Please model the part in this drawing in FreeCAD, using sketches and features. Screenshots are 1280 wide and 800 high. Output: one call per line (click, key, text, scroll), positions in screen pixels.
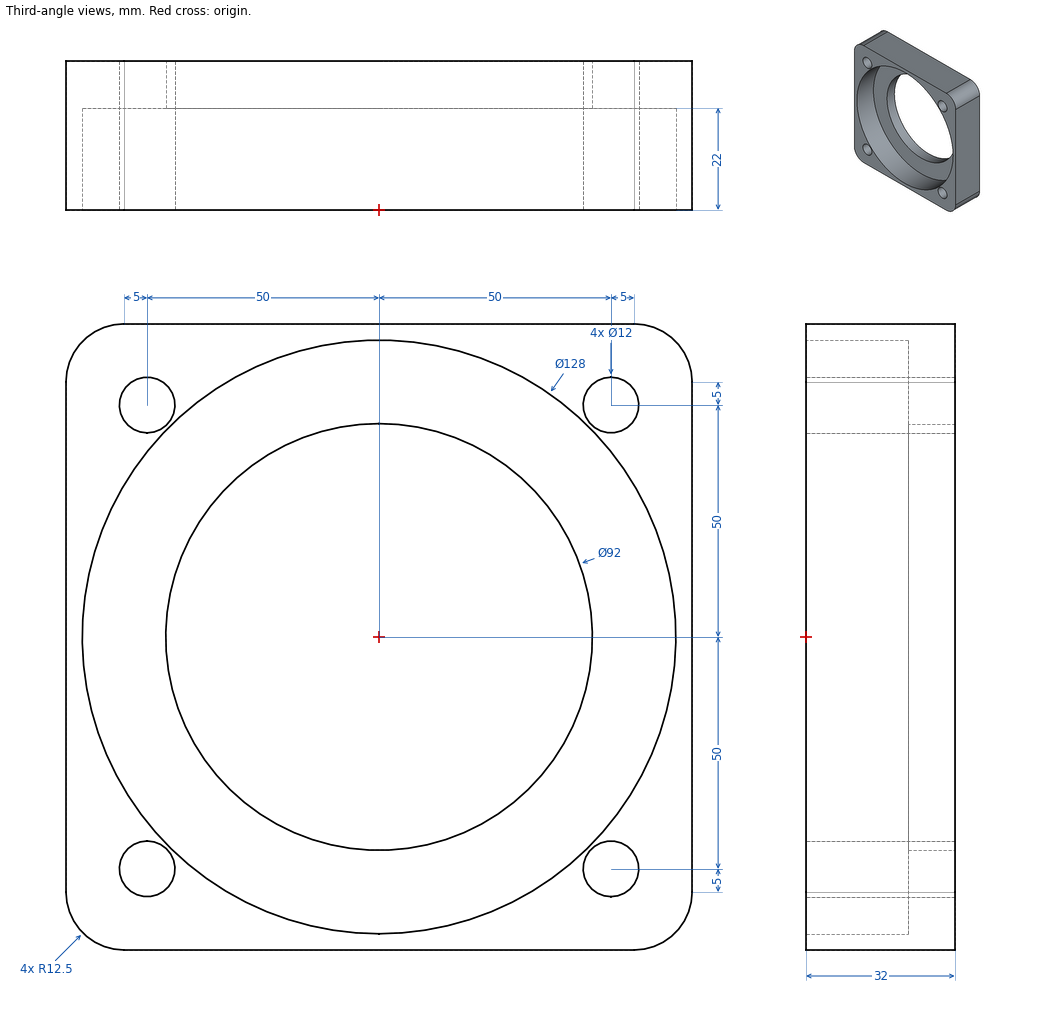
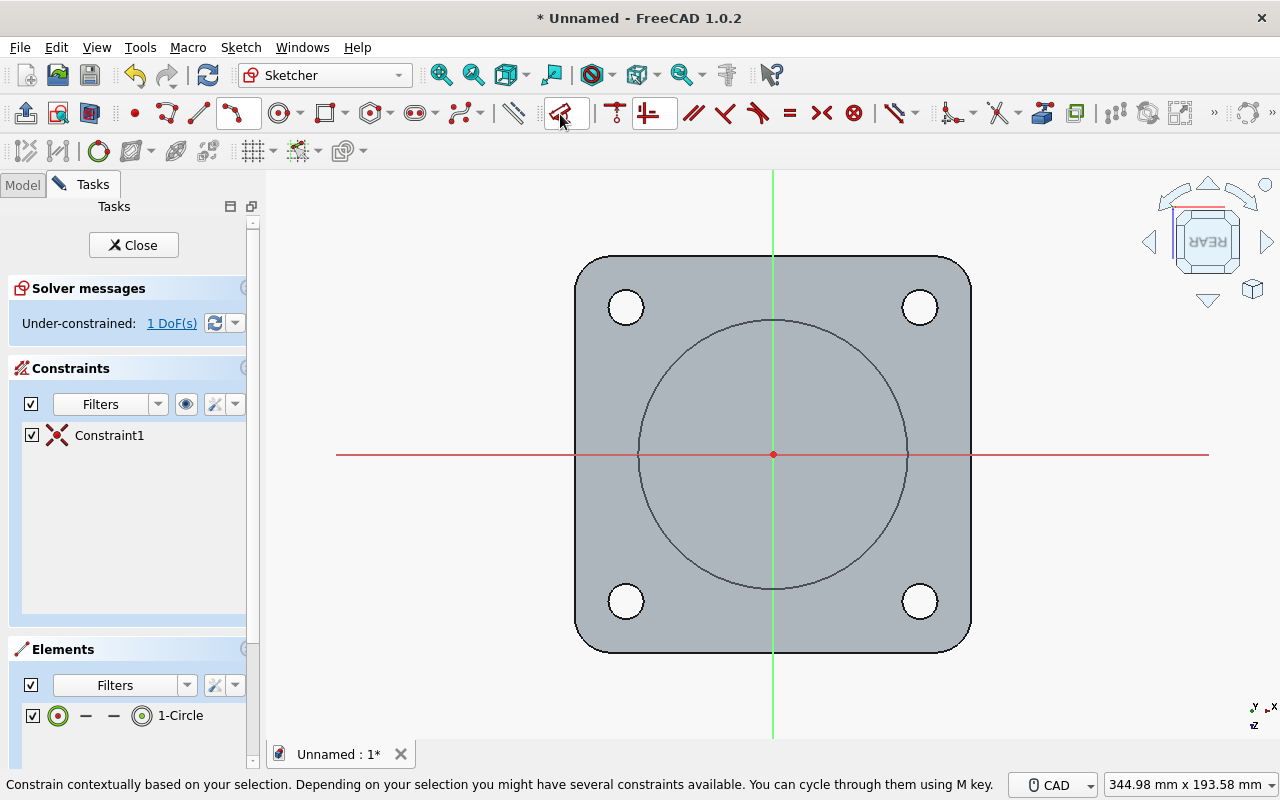
click(868, 359)
click(891, 336)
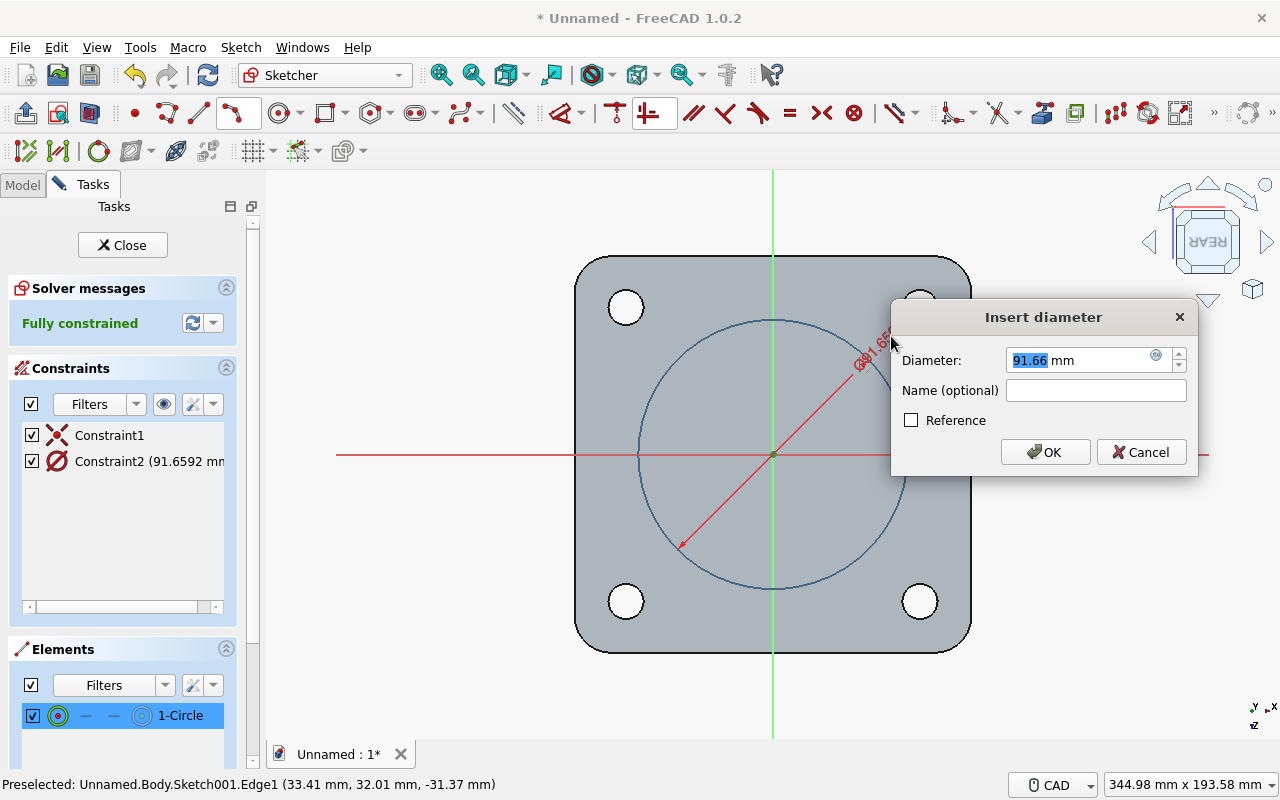
text(92)
key(Return)
key(Escape)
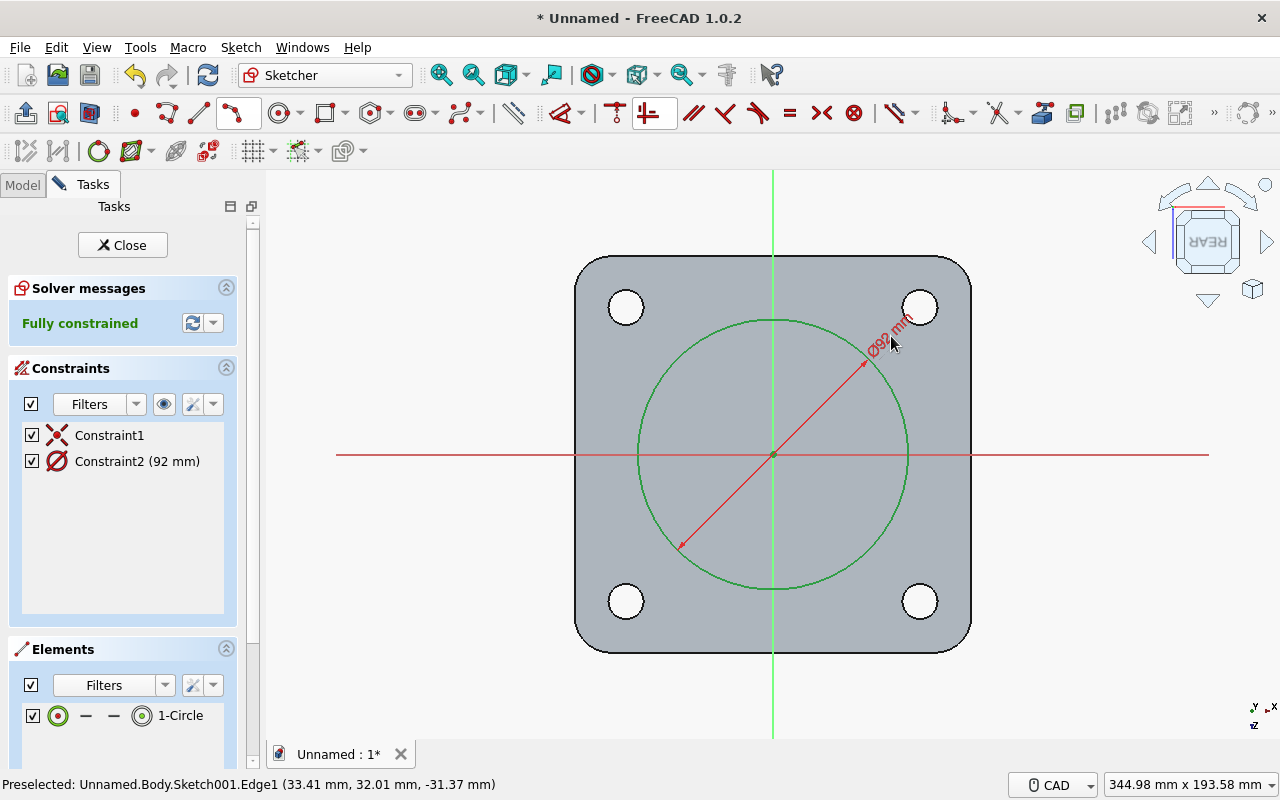
click(123, 245)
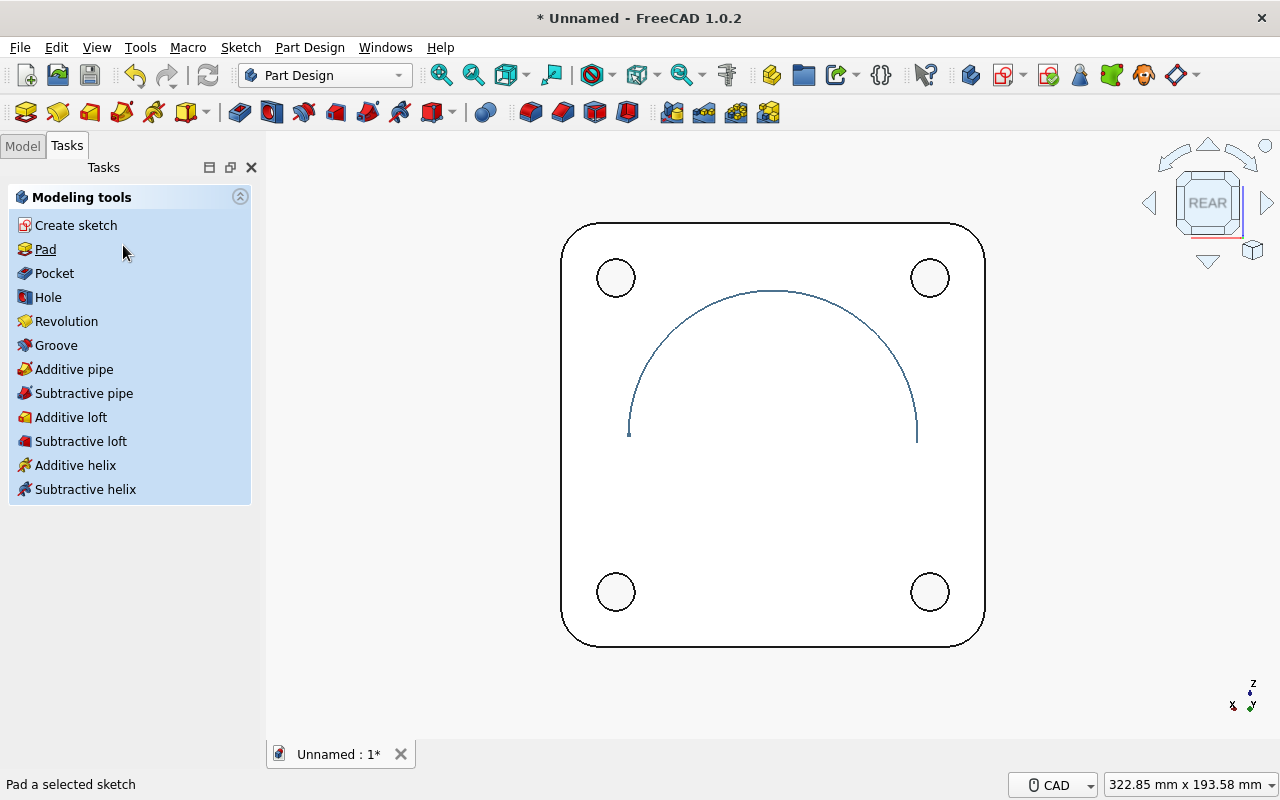
click(240, 112)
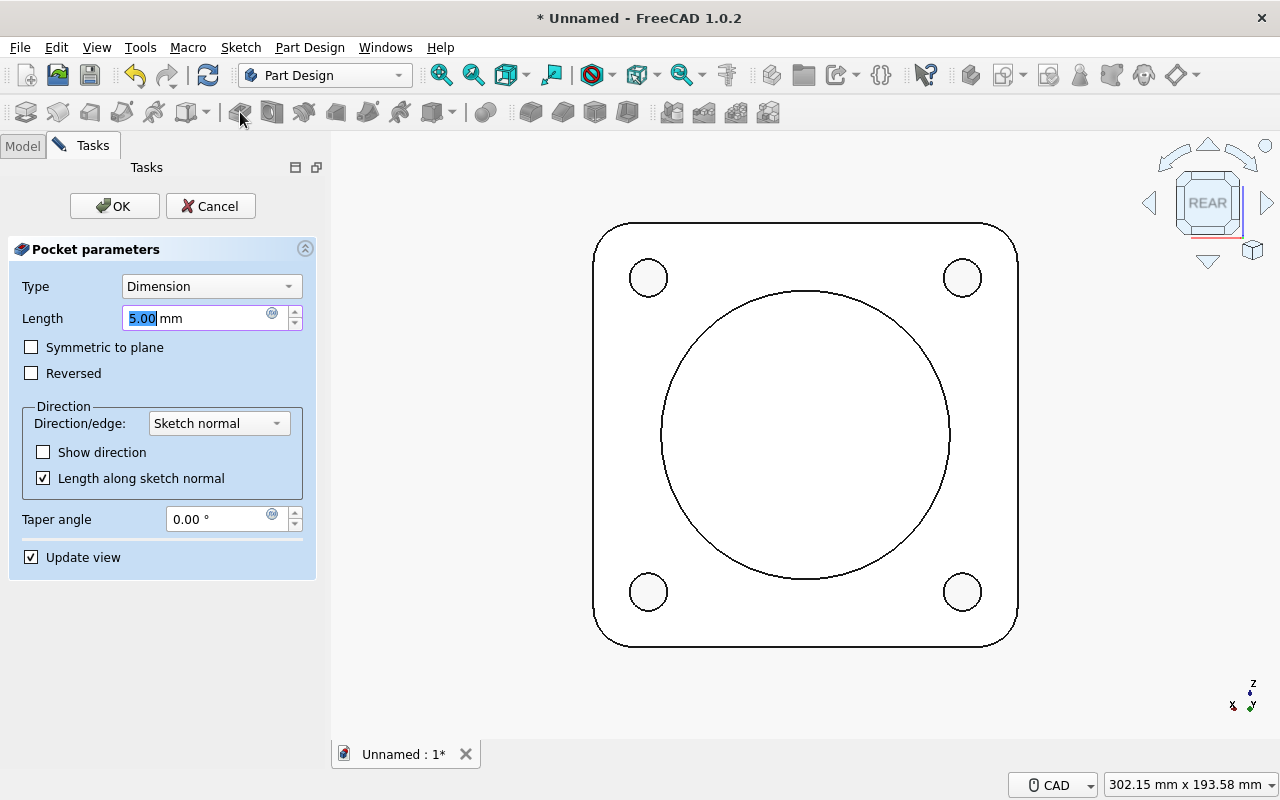
click(212, 286)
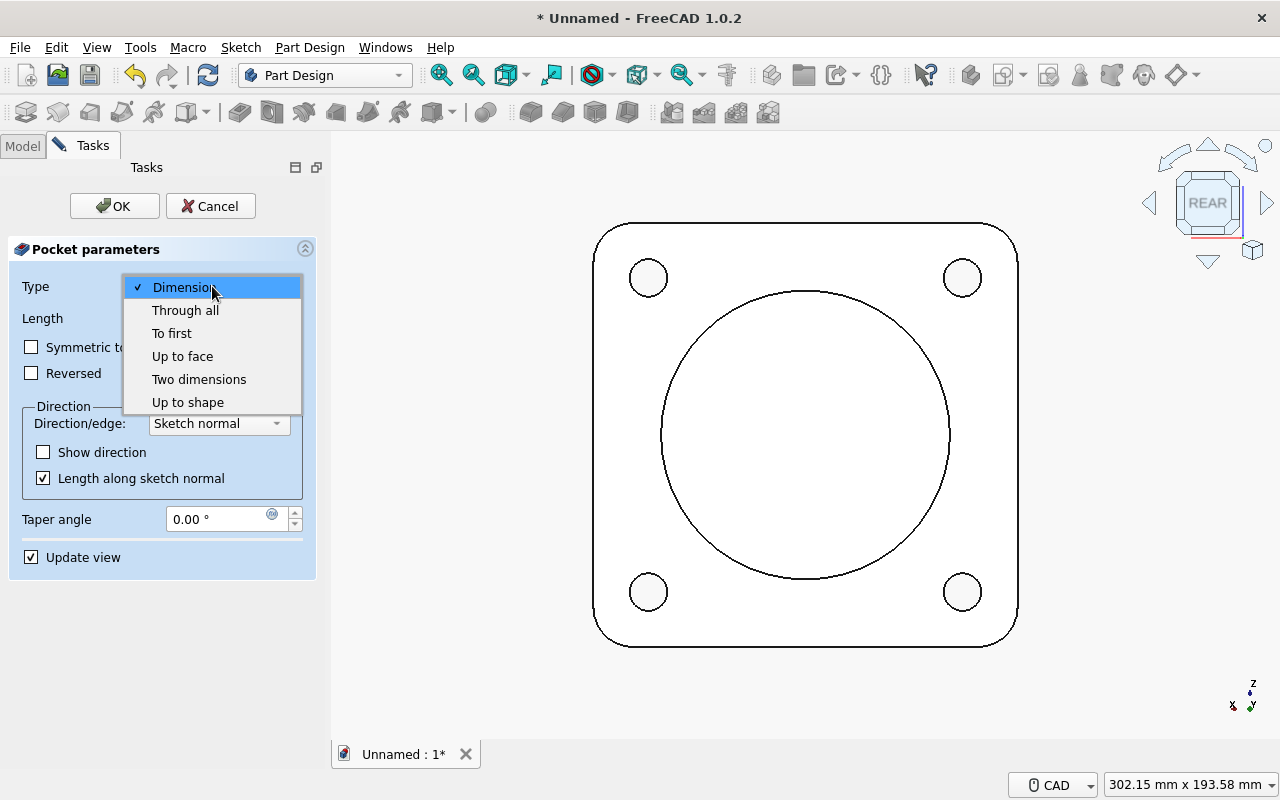
click(212, 334)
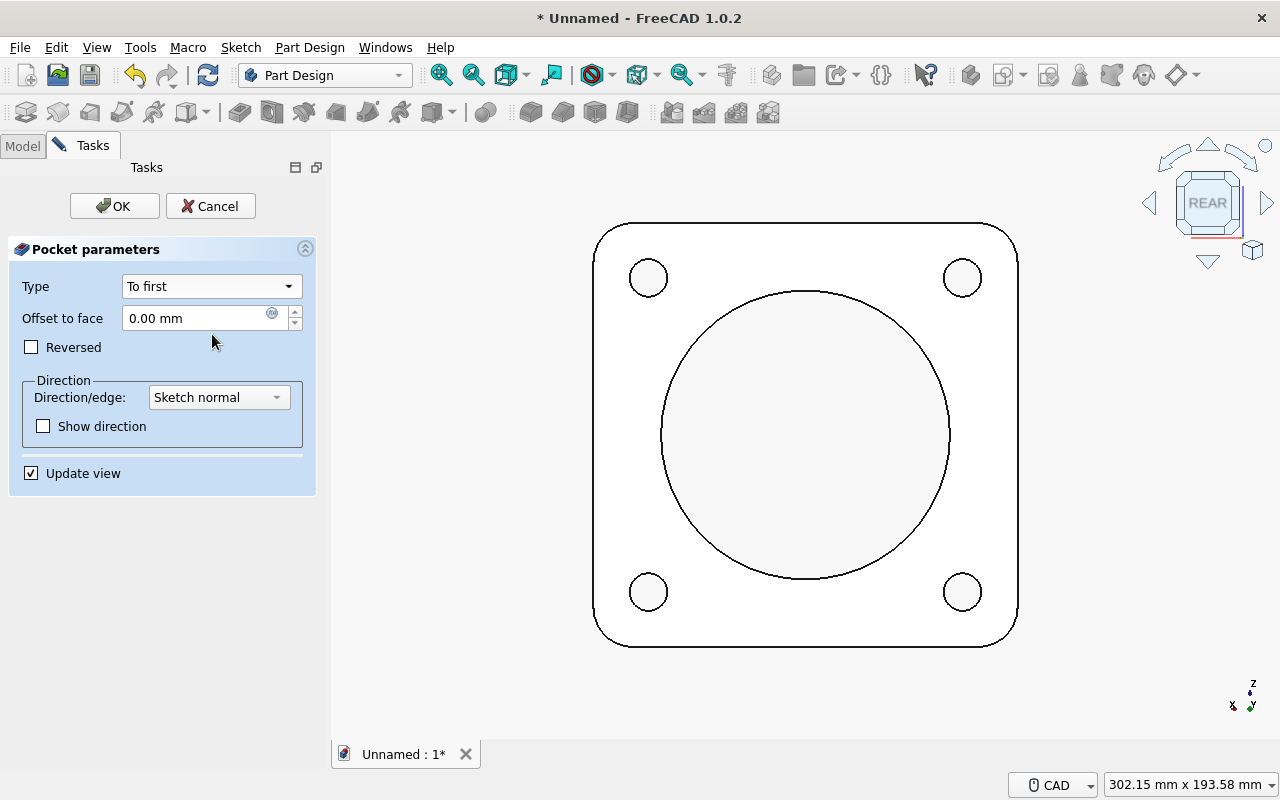
click(115, 206)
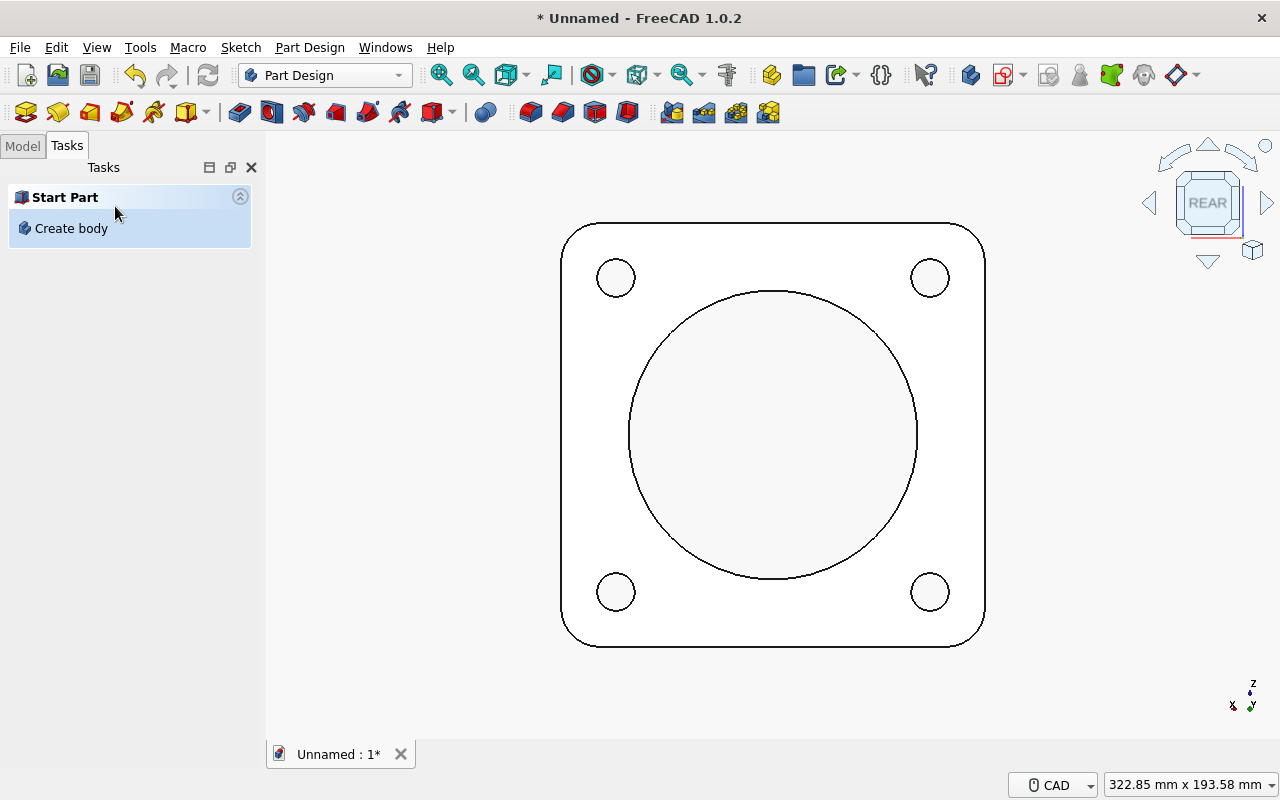
click(1004, 76)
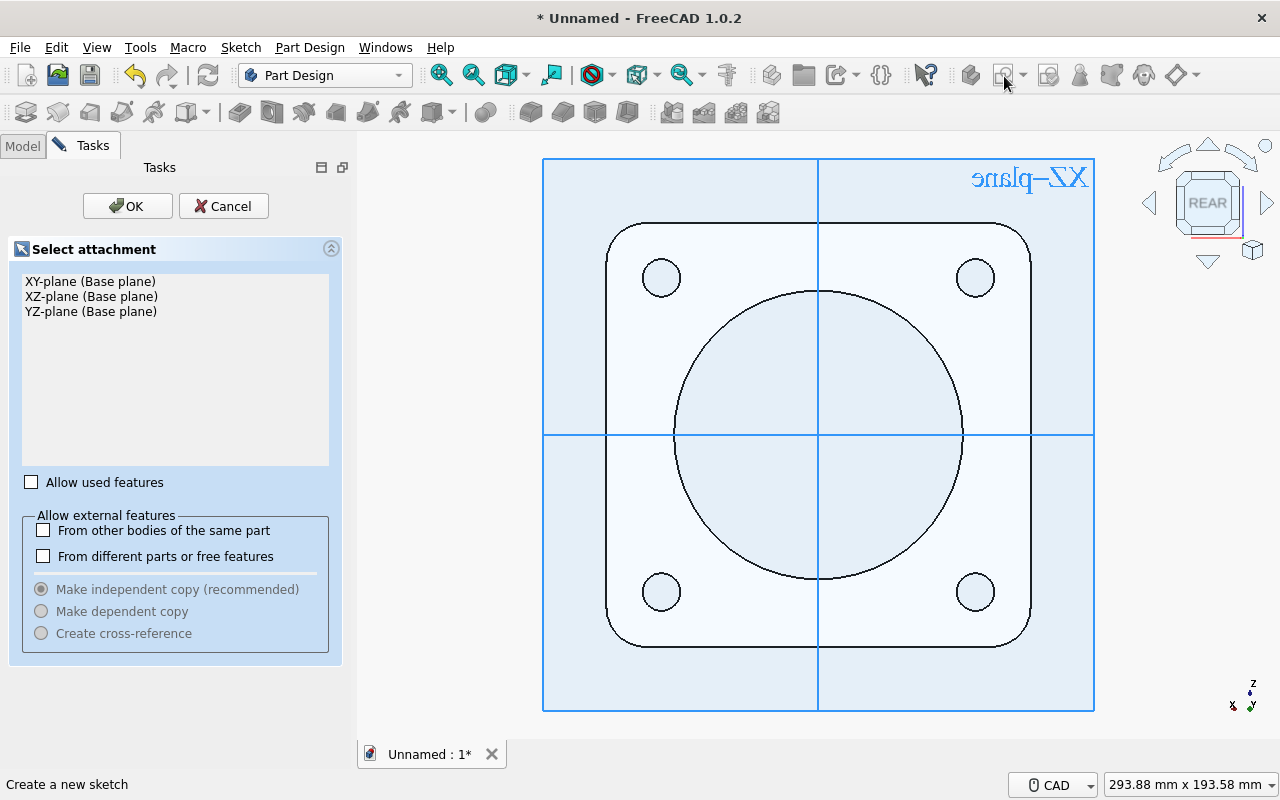
click(82, 296)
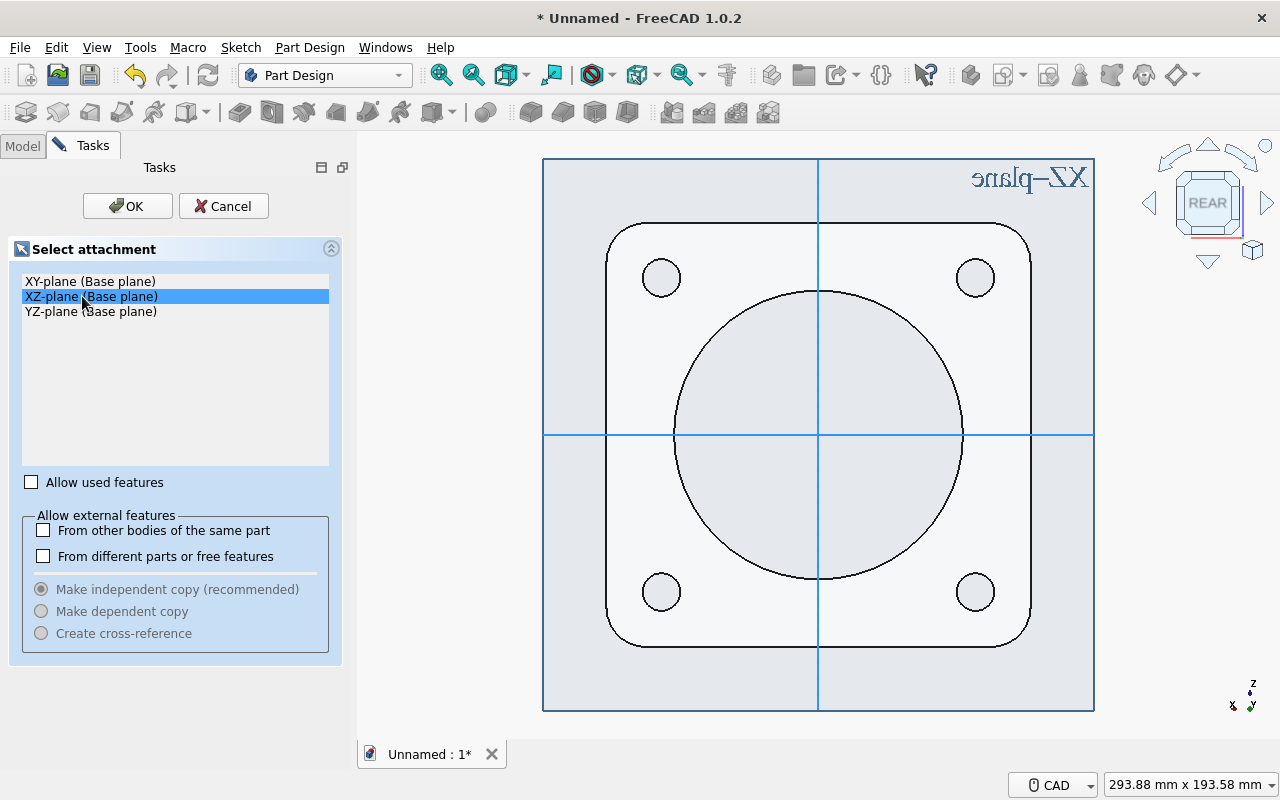
click(128, 206)